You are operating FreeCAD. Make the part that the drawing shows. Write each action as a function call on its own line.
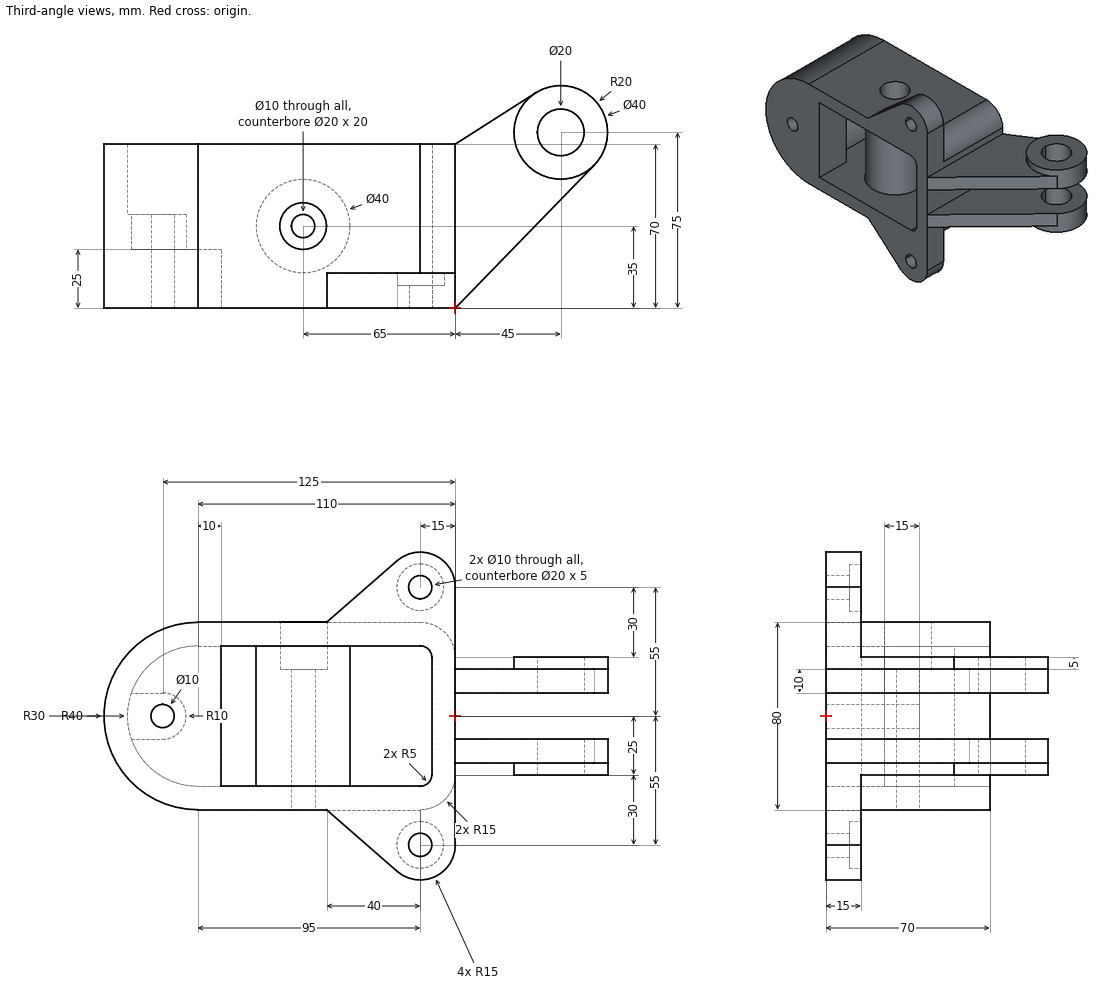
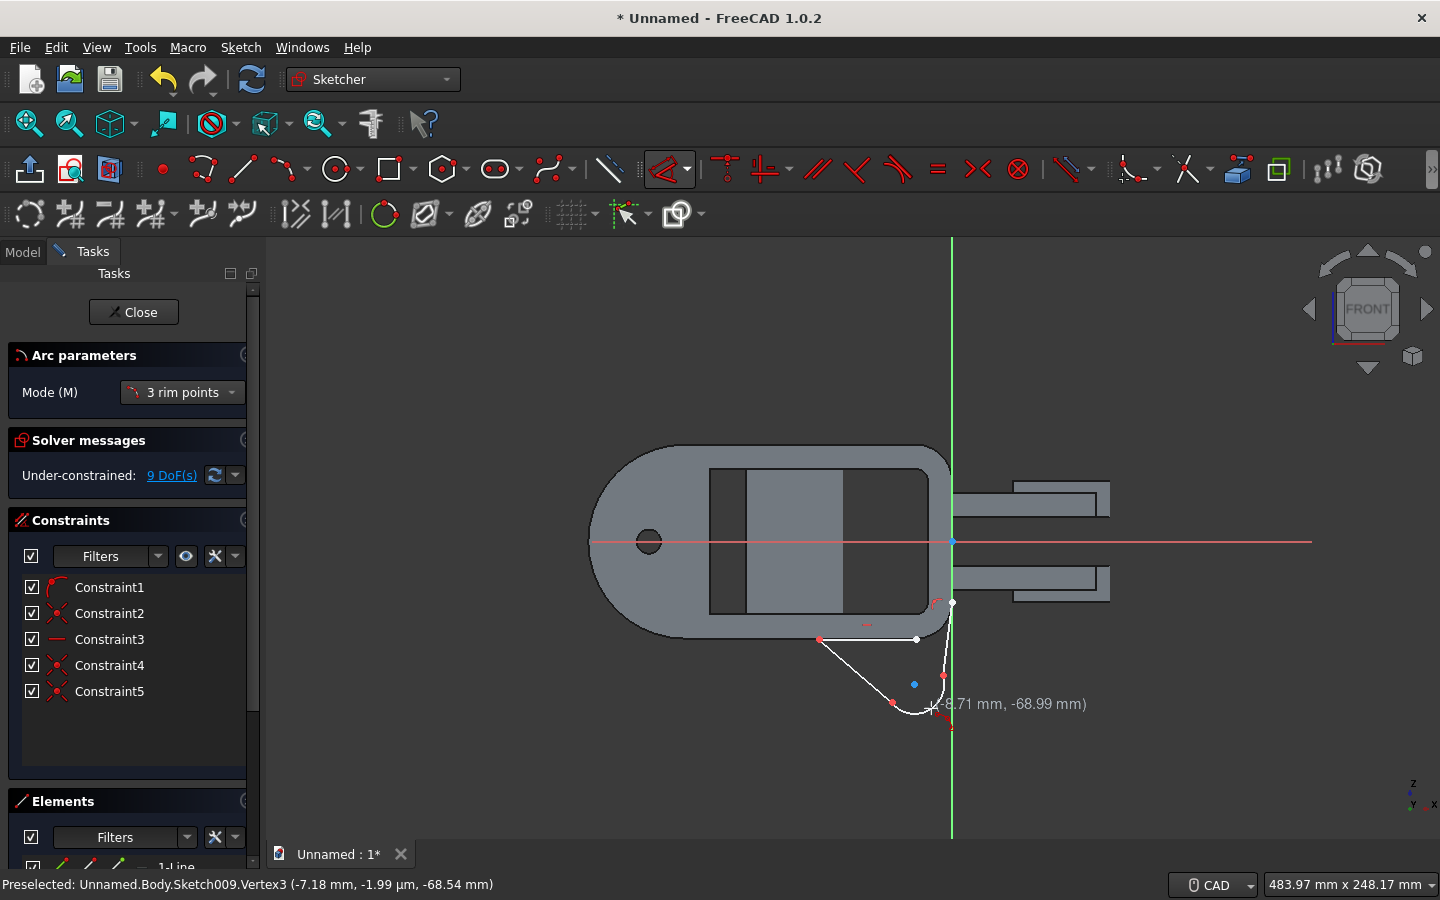
click(916, 640)
click(952, 603)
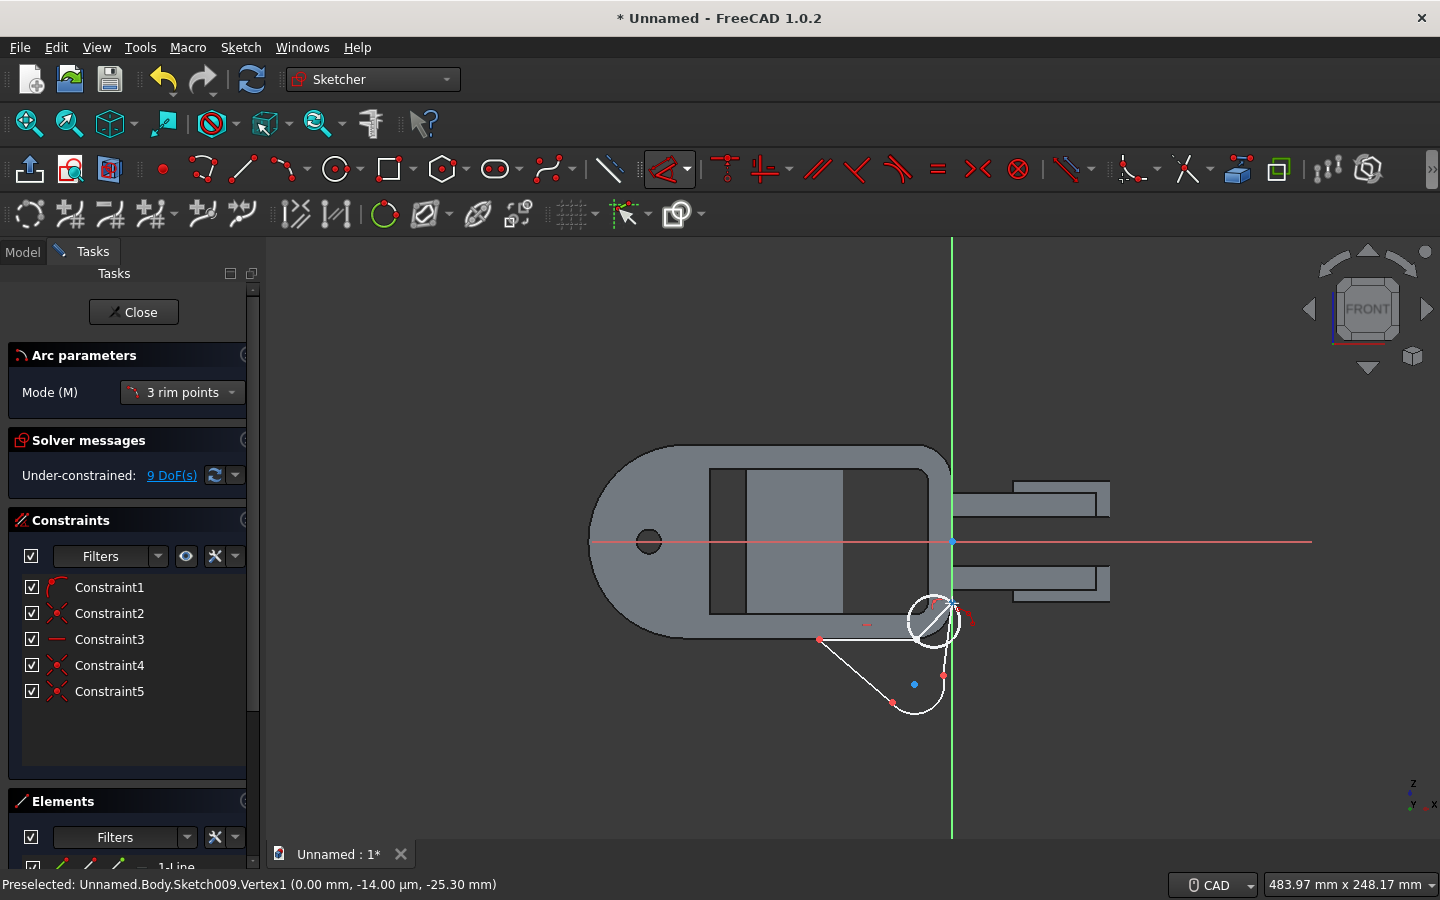
scroll(941, 628, up, 2)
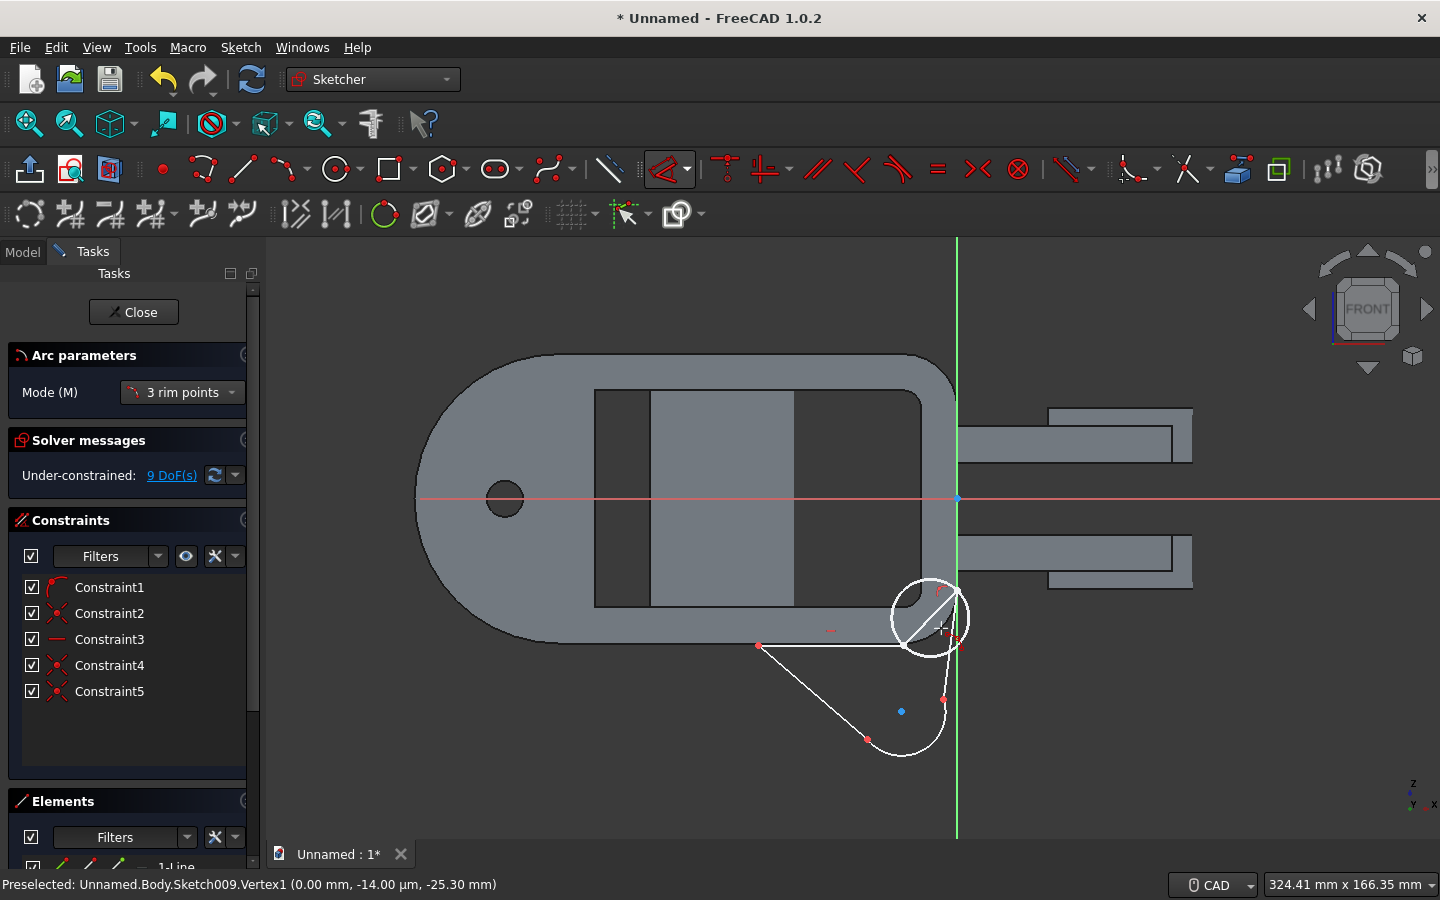
click(941, 628)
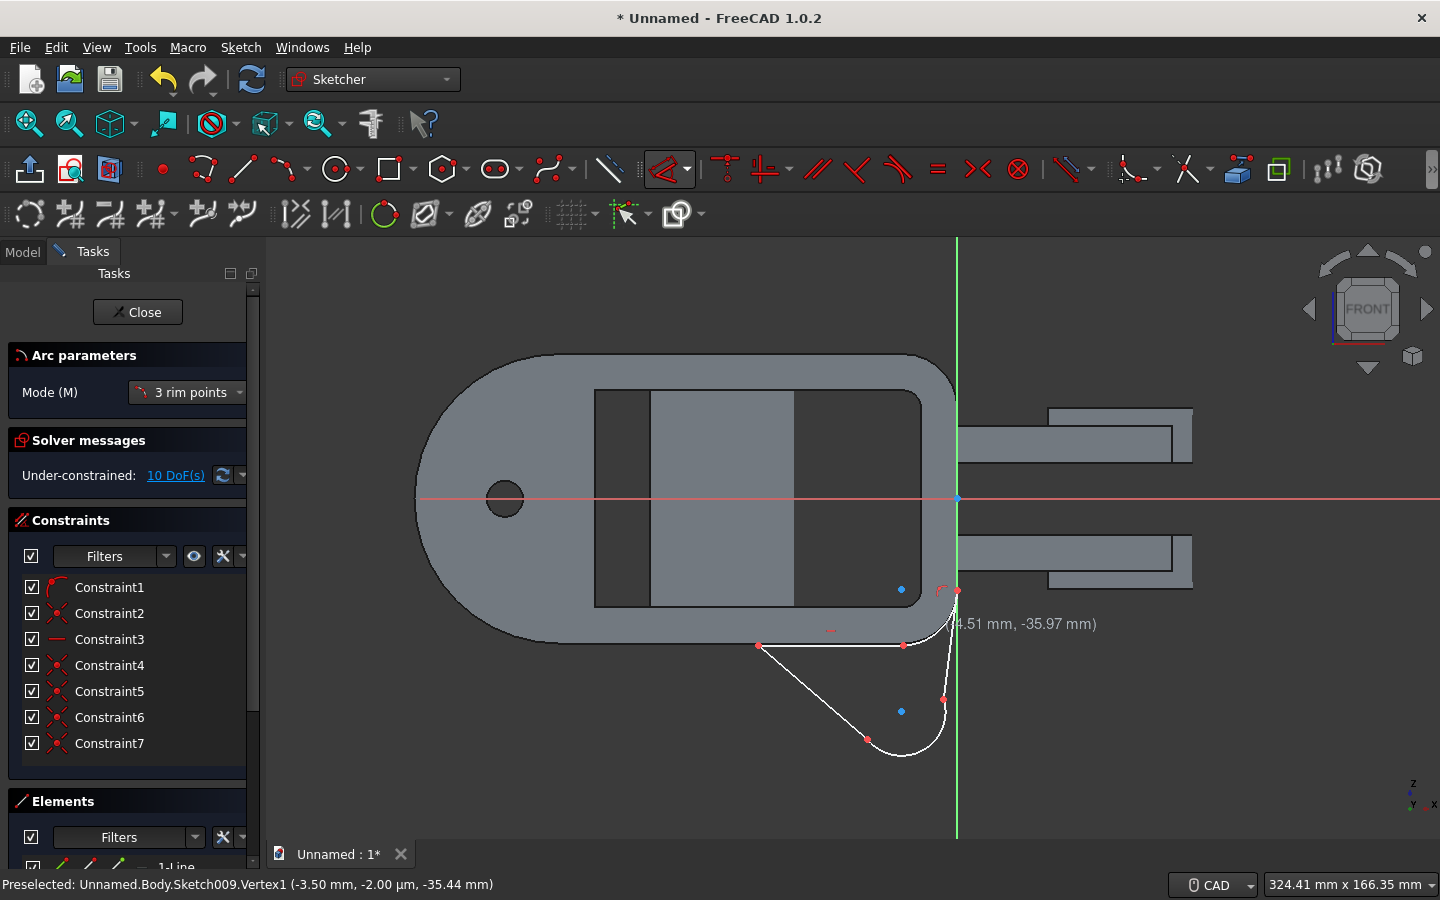
key(g)
key(l)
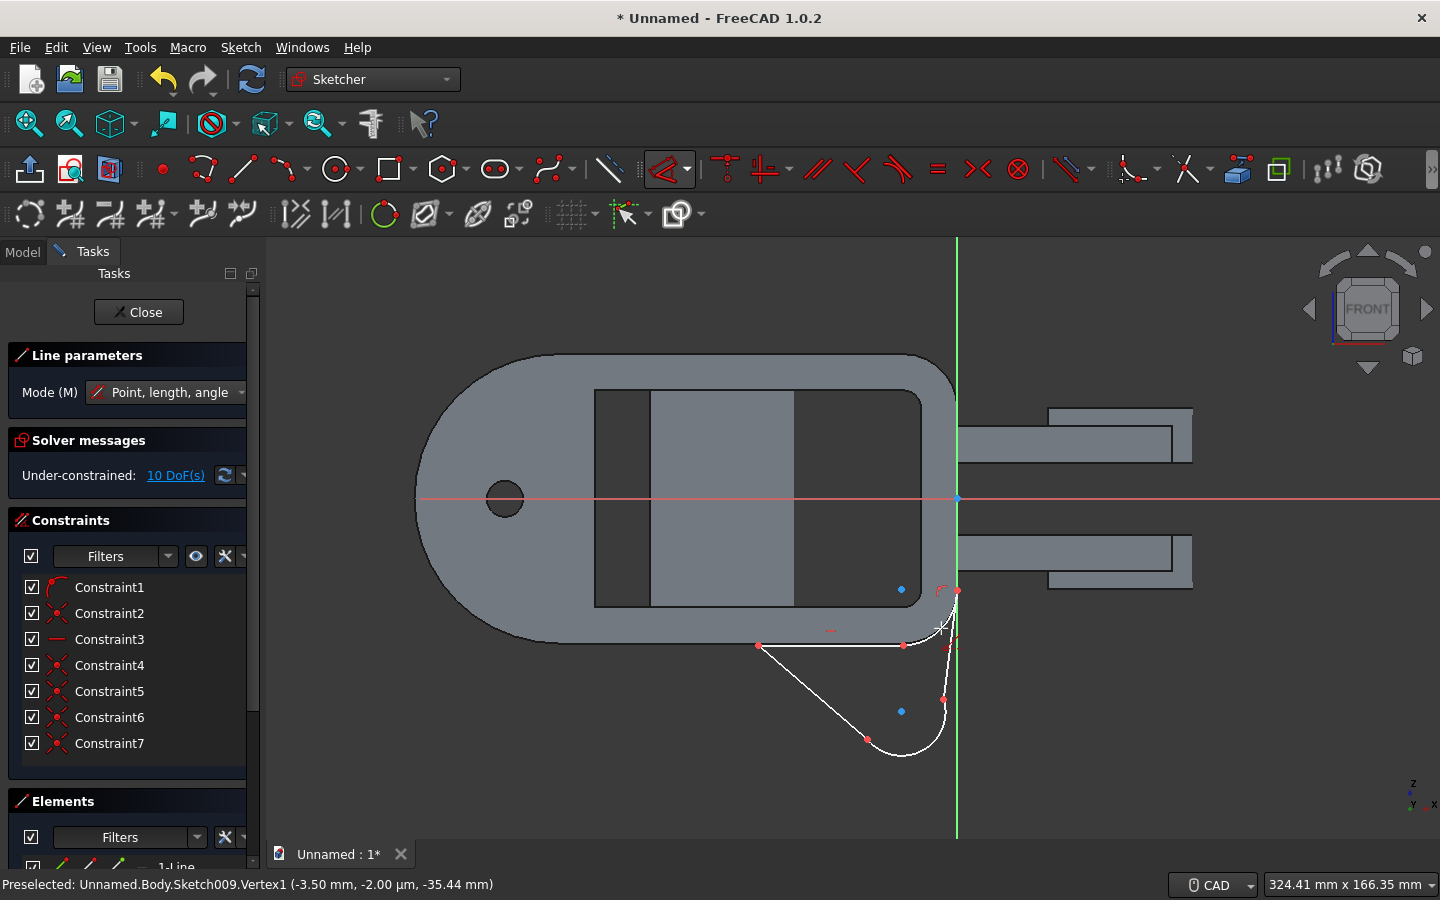
click(957, 300)
click(948, 408)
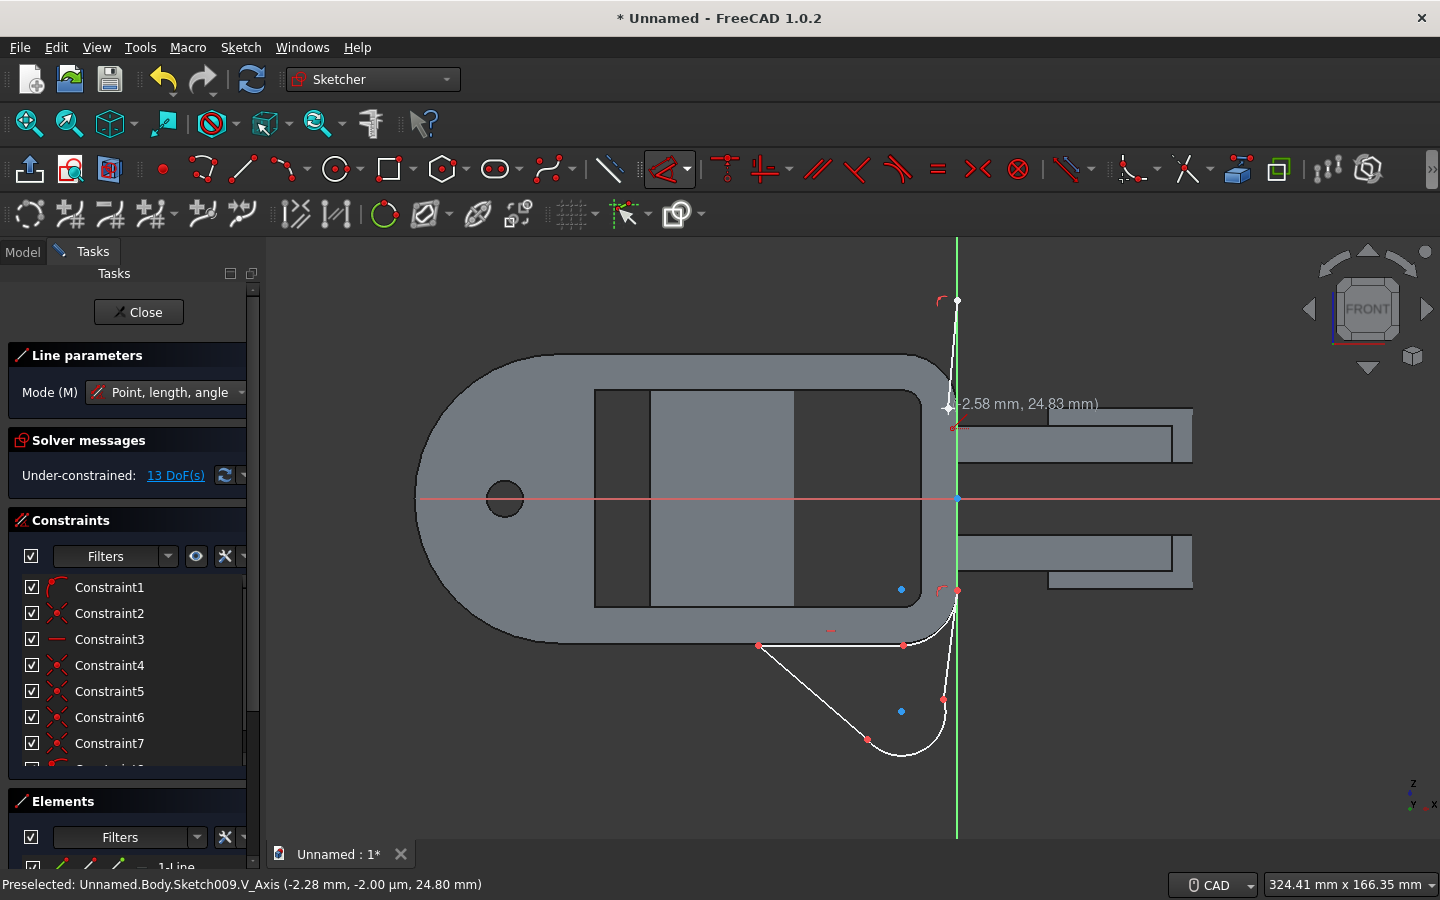
key(g)
key(m)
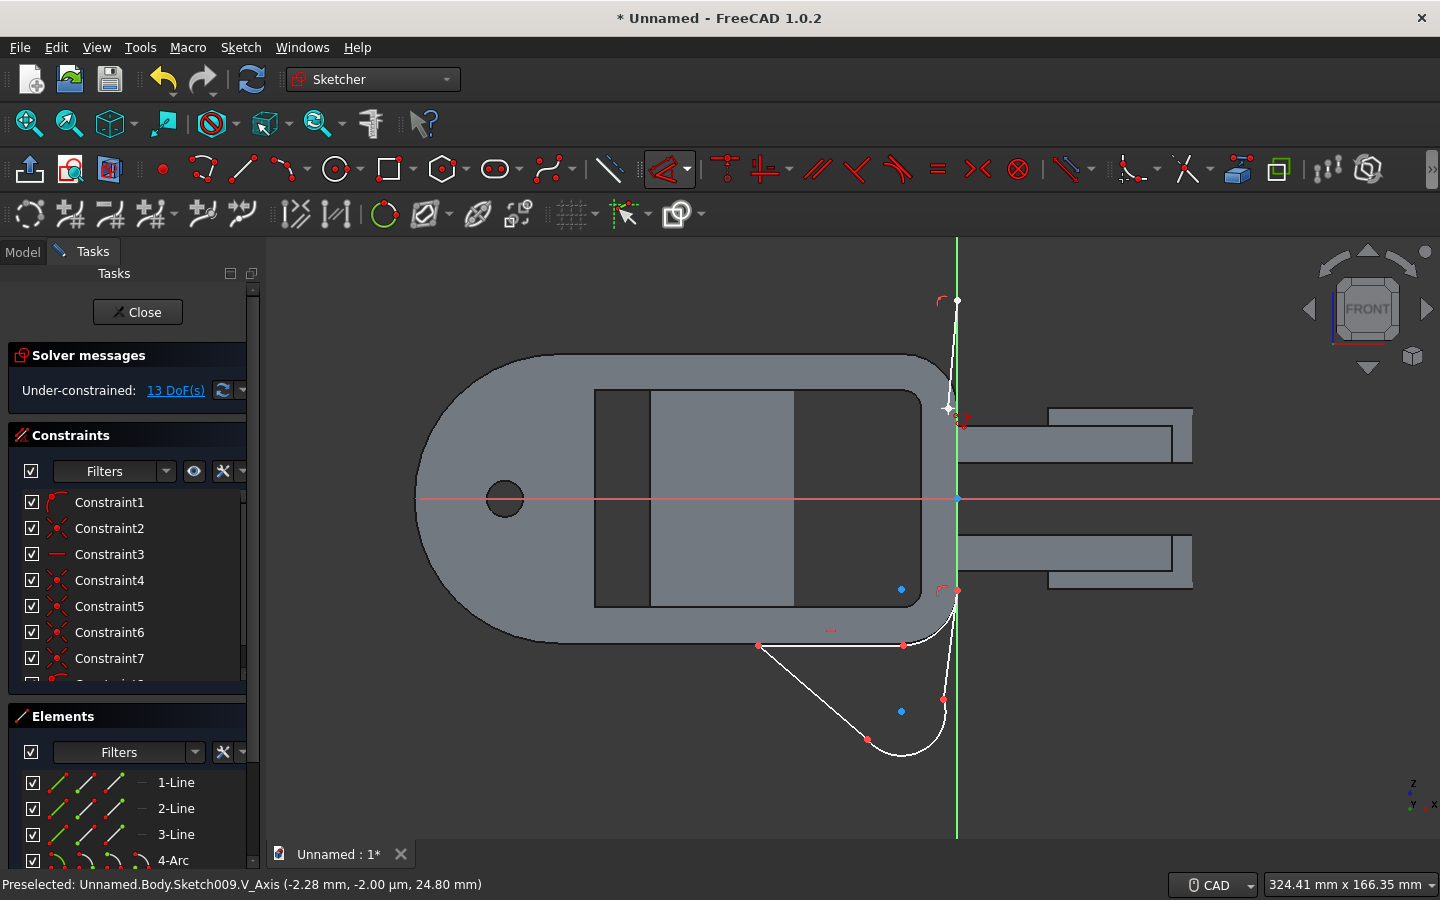
click(903, 354)
click(758, 354)